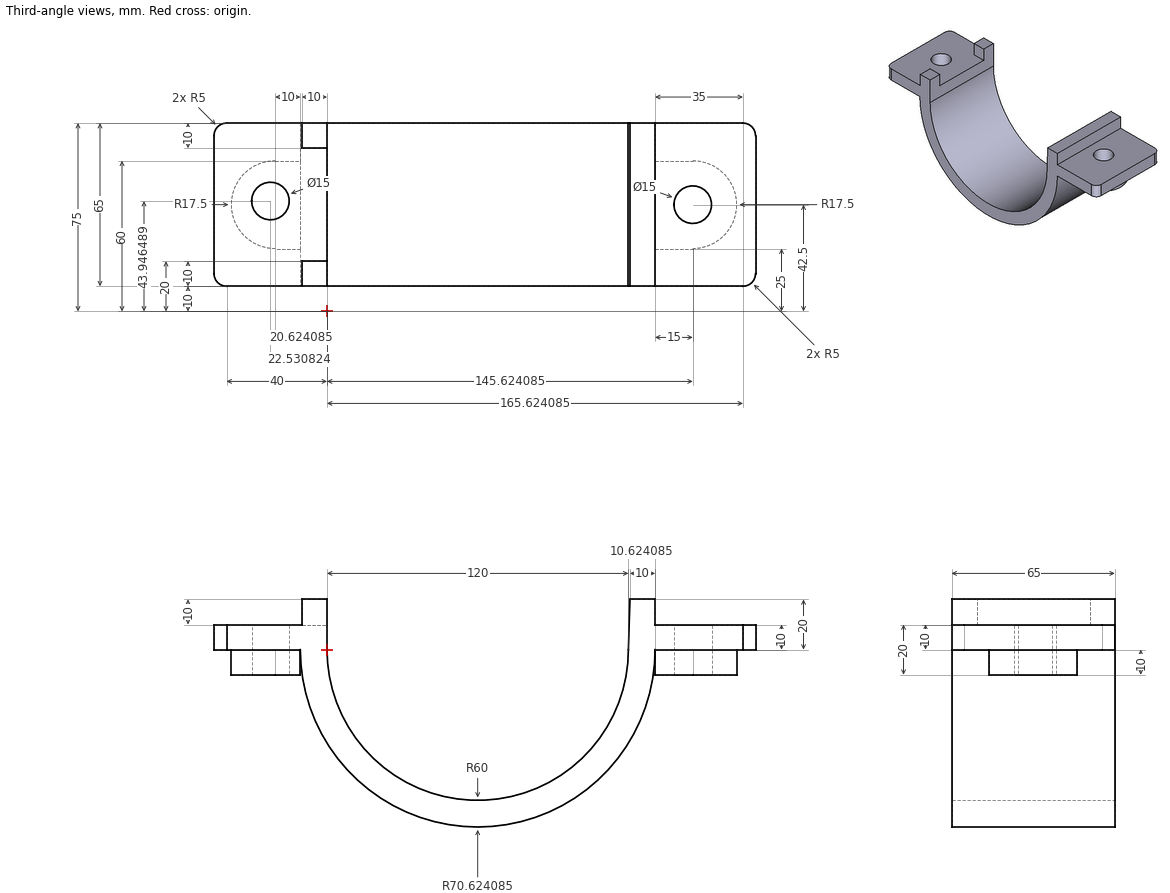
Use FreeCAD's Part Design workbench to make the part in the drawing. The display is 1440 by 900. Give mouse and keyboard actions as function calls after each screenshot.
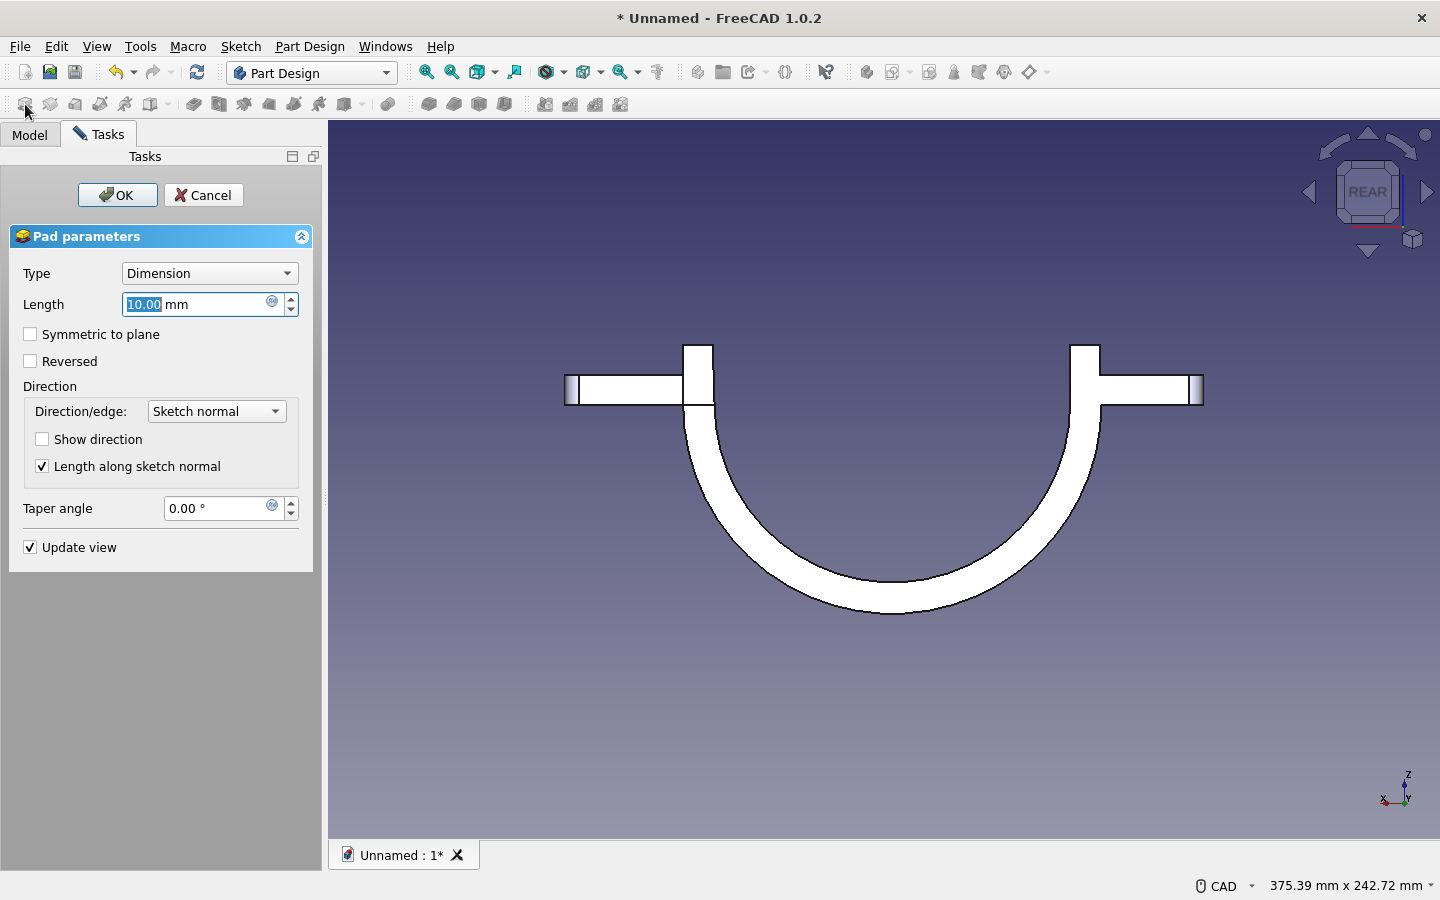
text(65)
key(Tab)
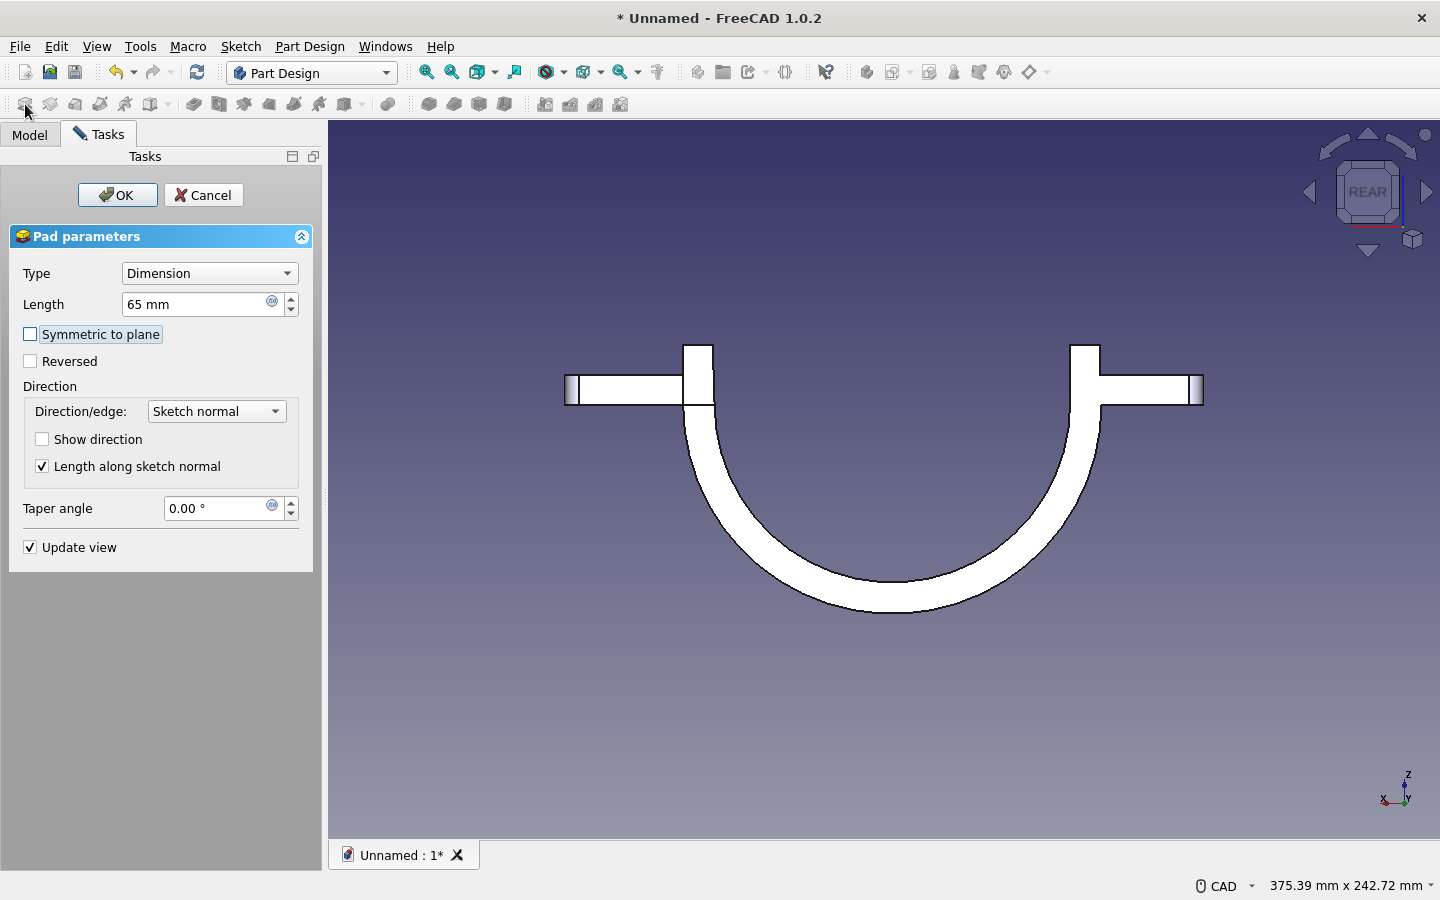
click(31, 361)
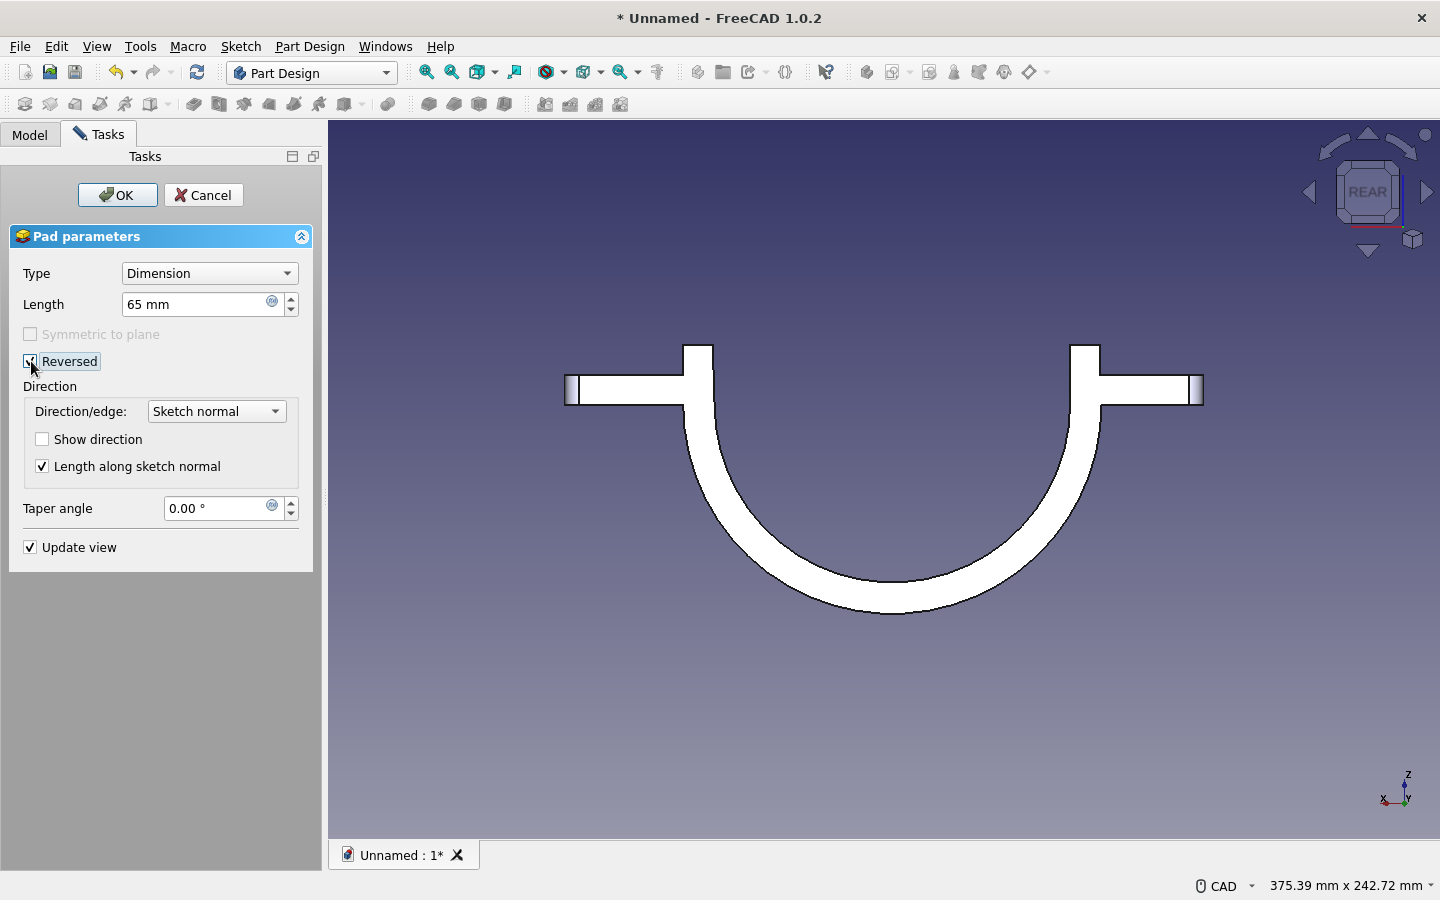
click(118, 195)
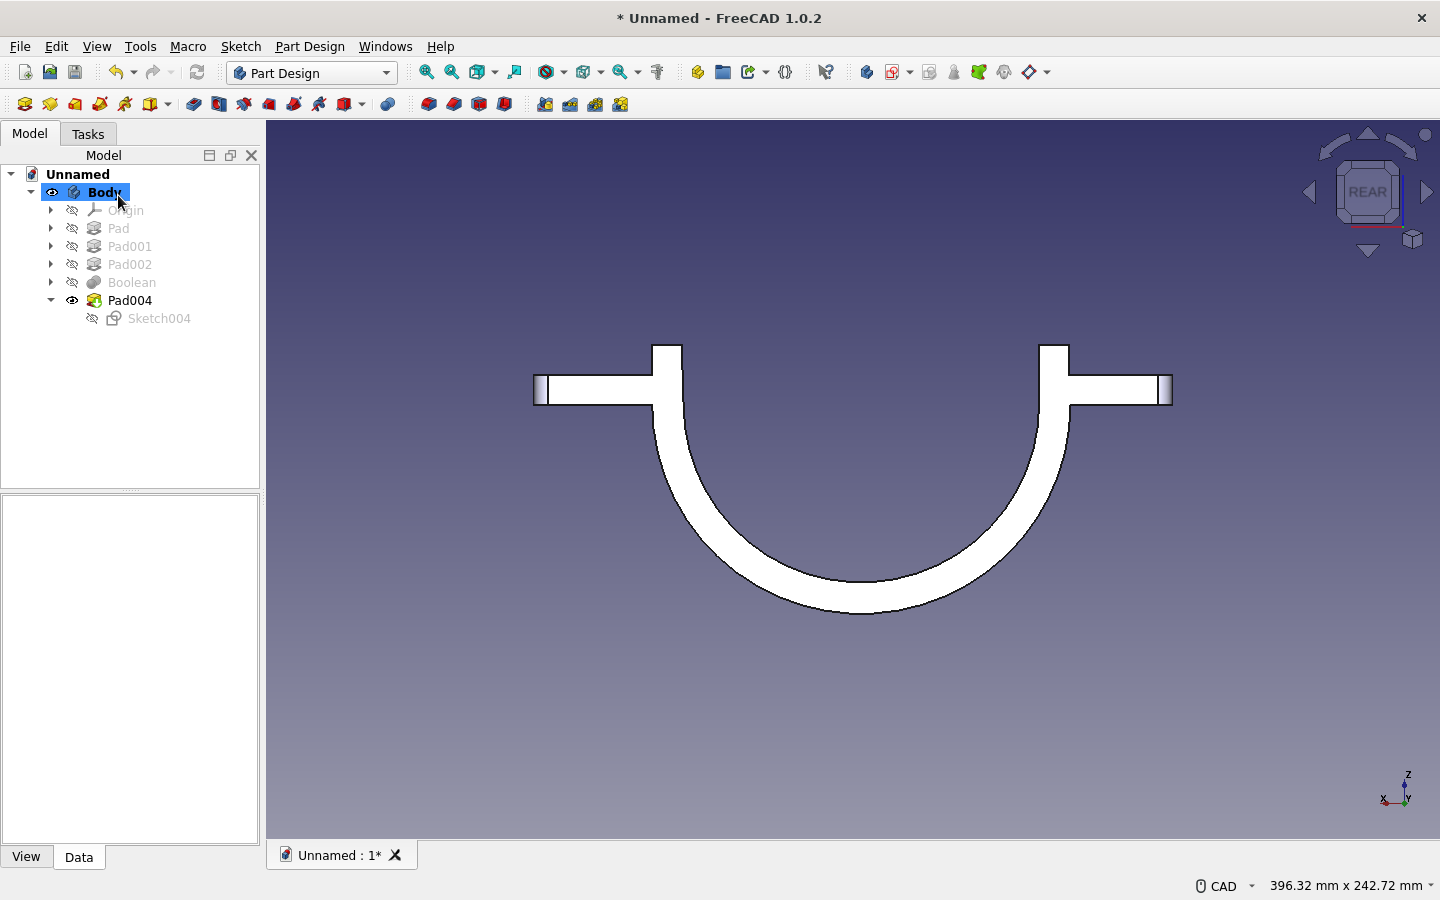
click(892, 72)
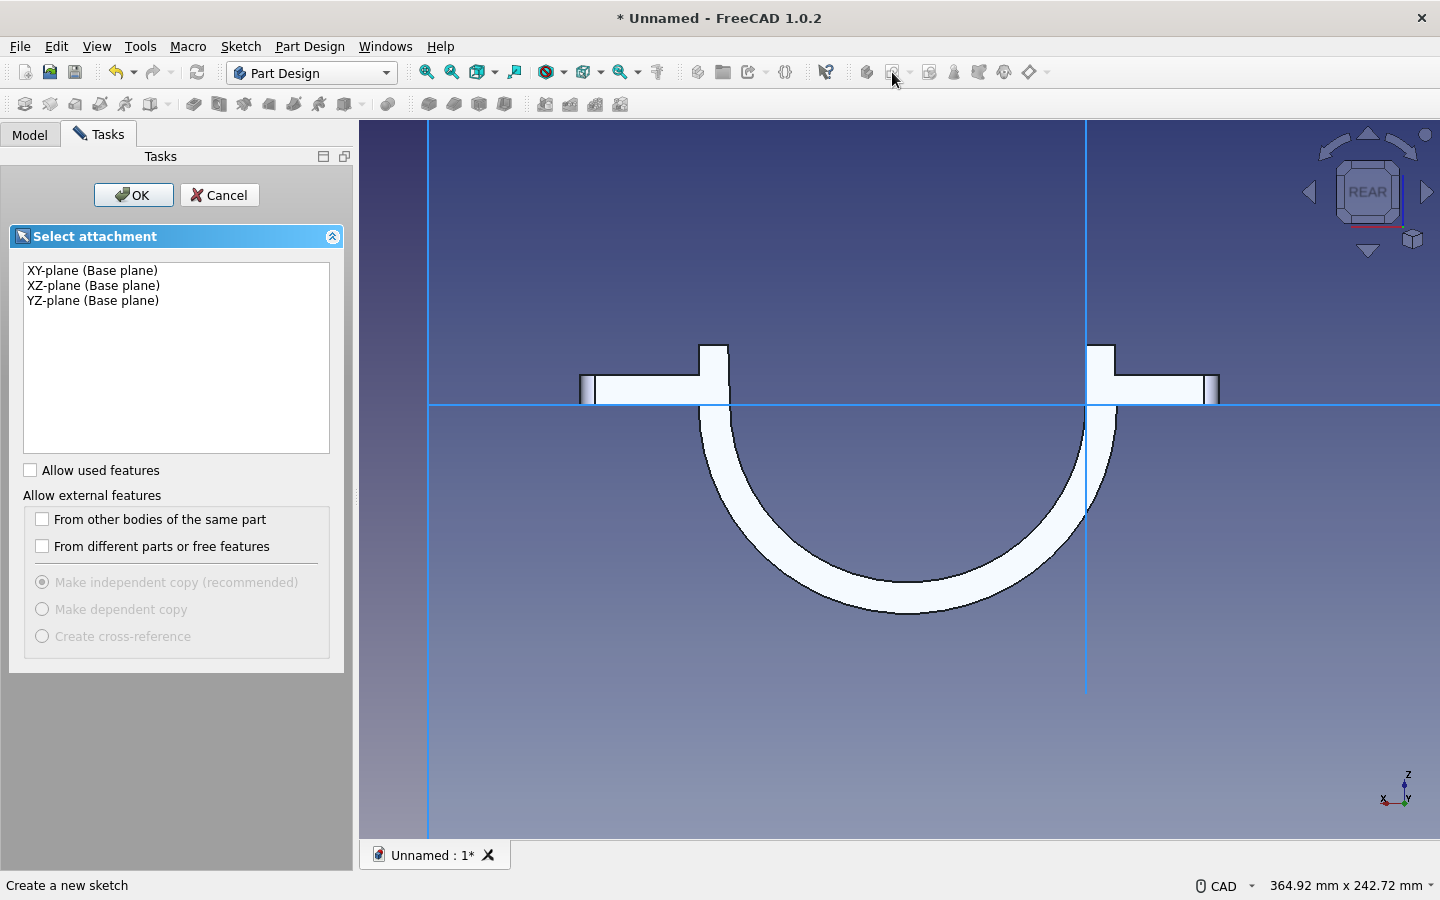
click(84, 270)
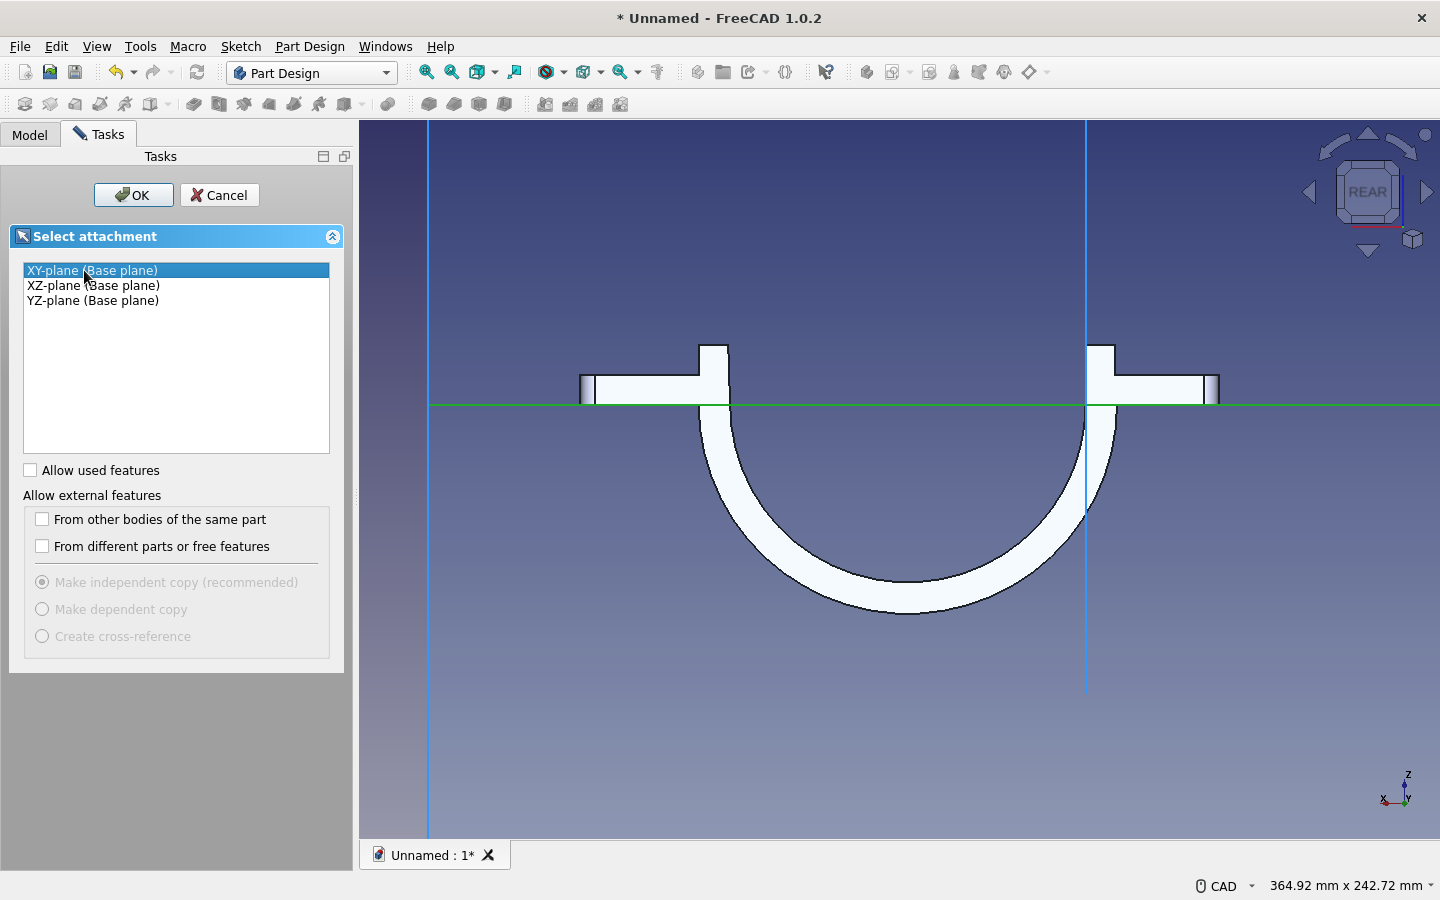
click(134, 195)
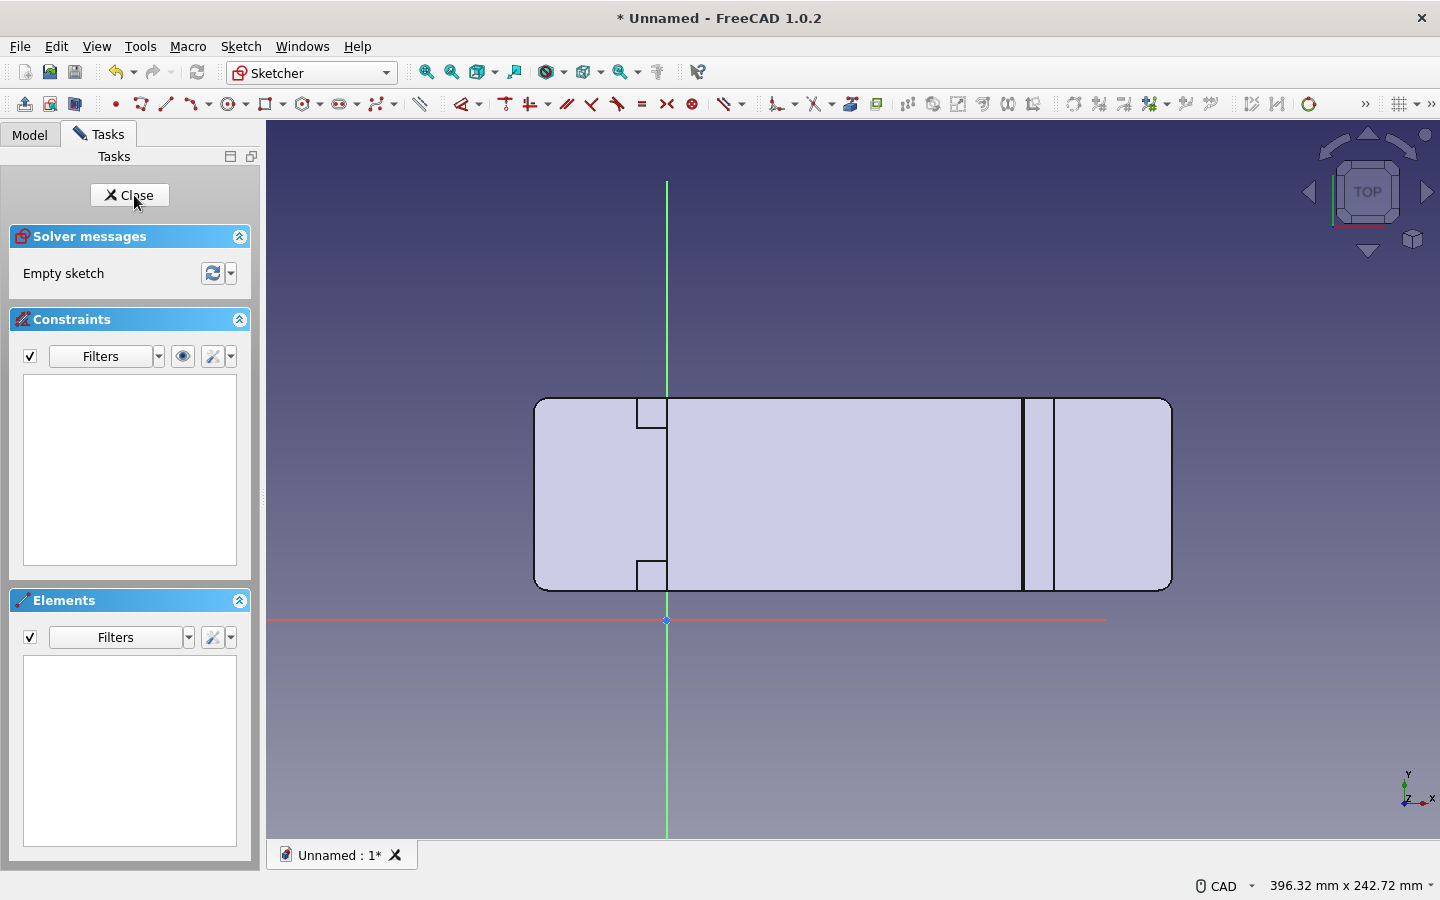
key(q)
key(s)